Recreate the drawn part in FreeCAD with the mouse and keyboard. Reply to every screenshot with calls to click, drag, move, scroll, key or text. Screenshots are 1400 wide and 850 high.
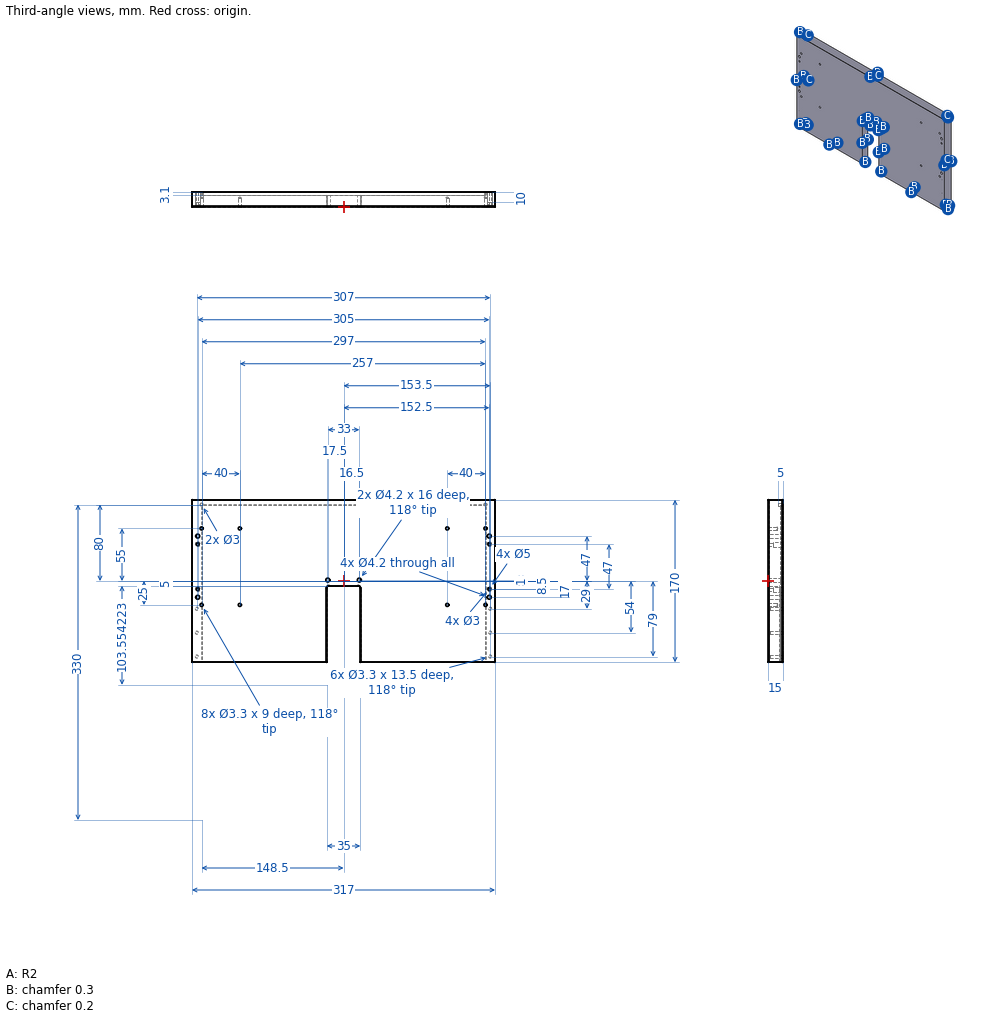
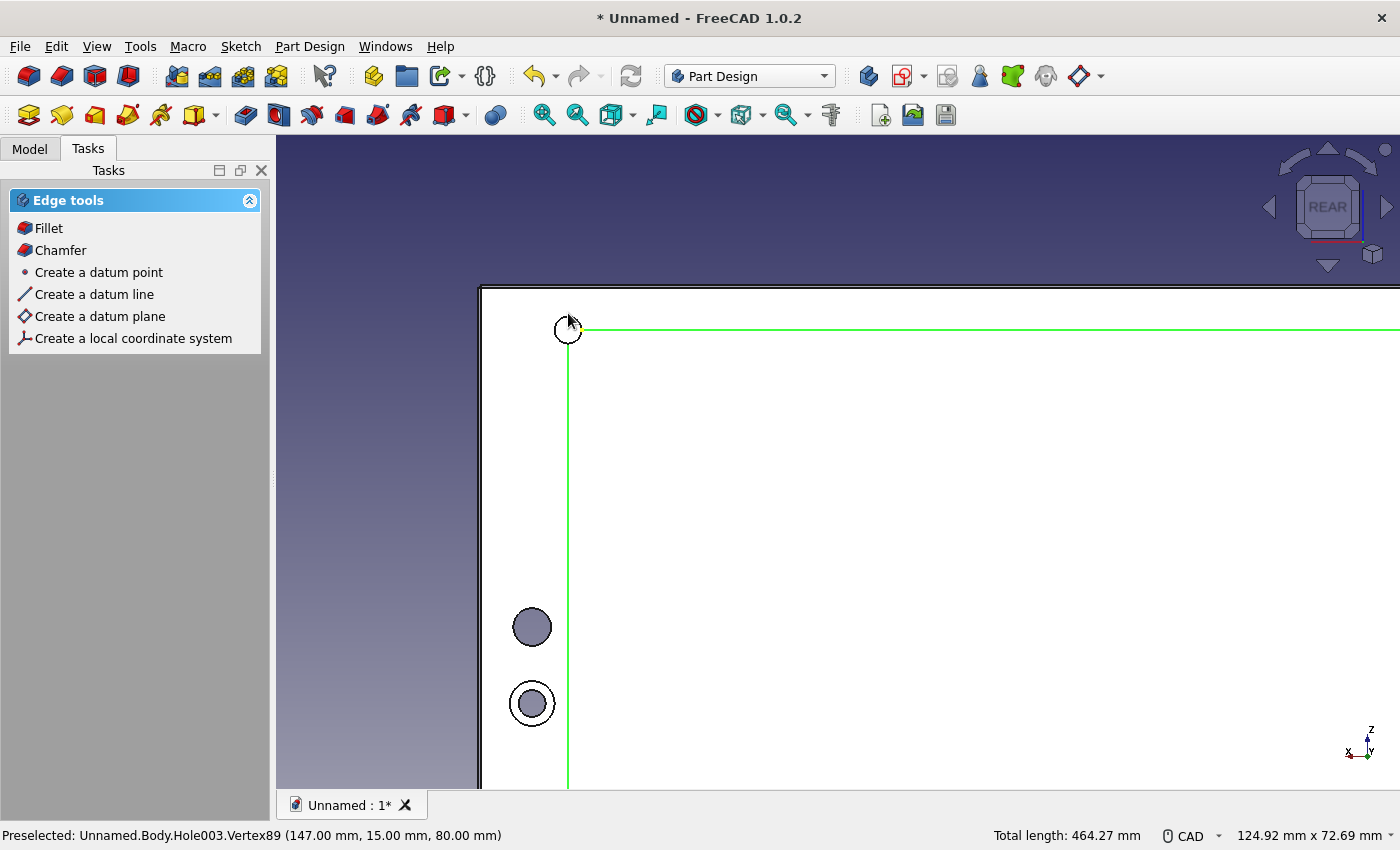
click(568, 316, ctrl)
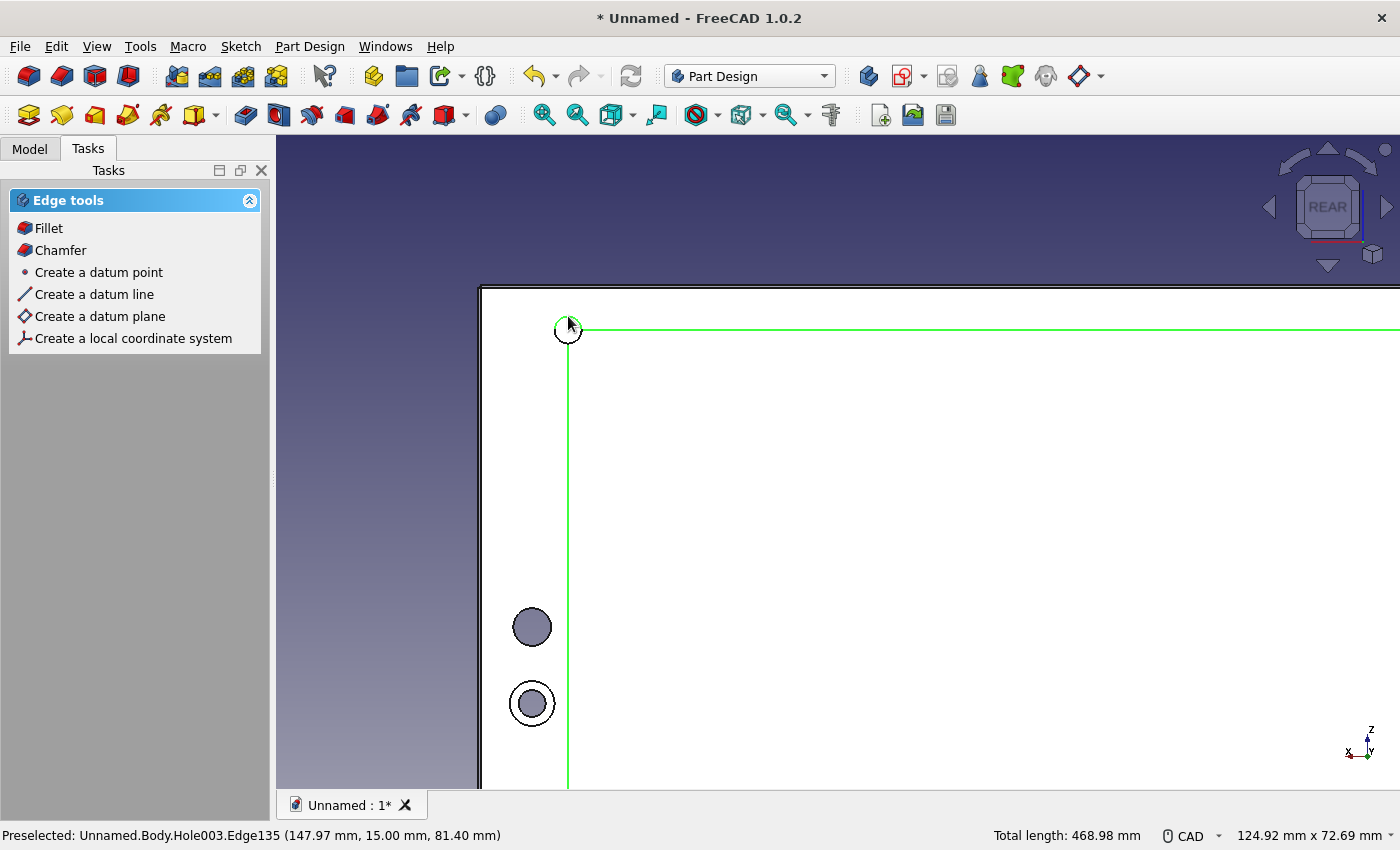
key(v)
key(f)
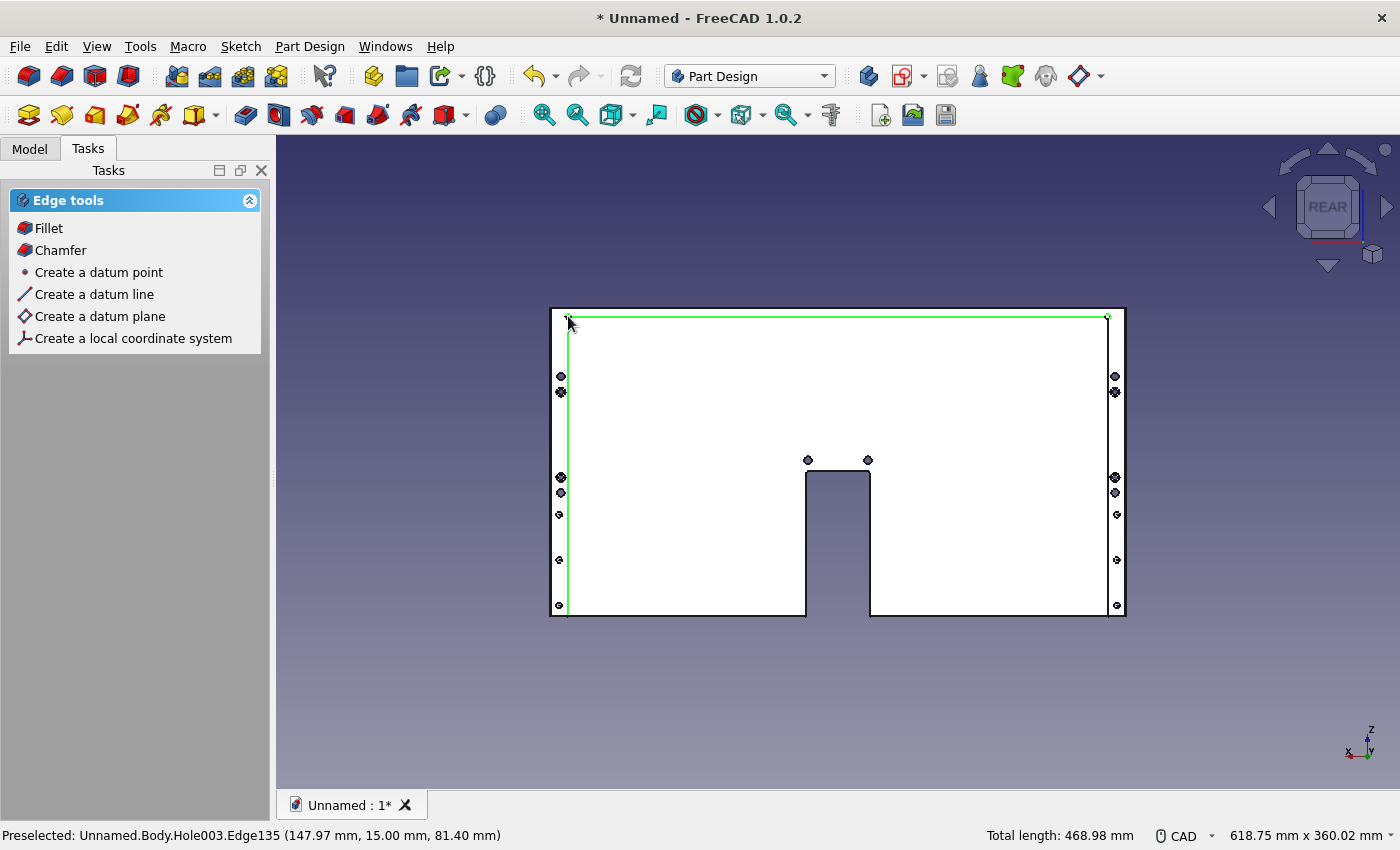
key(0)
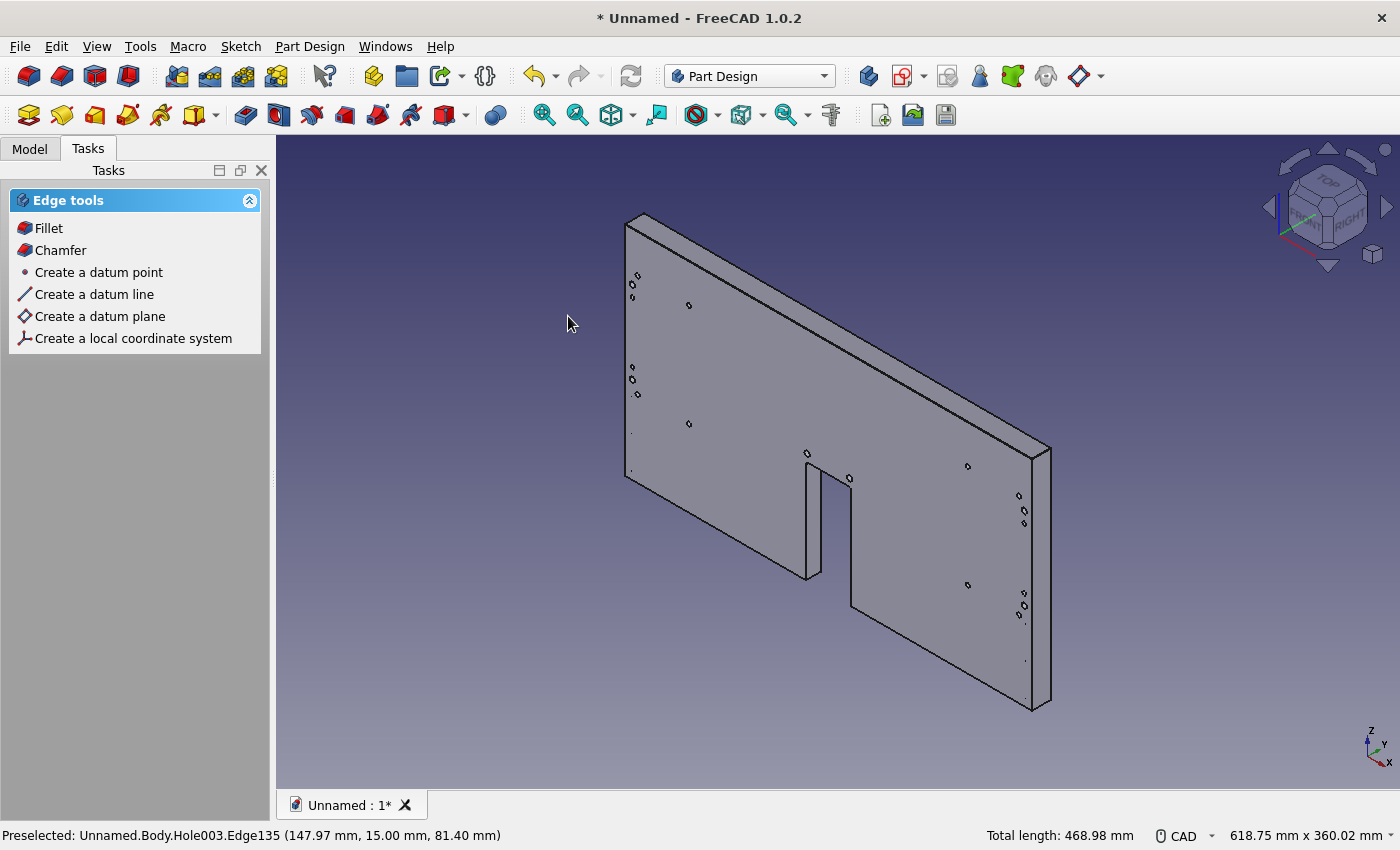
key(2)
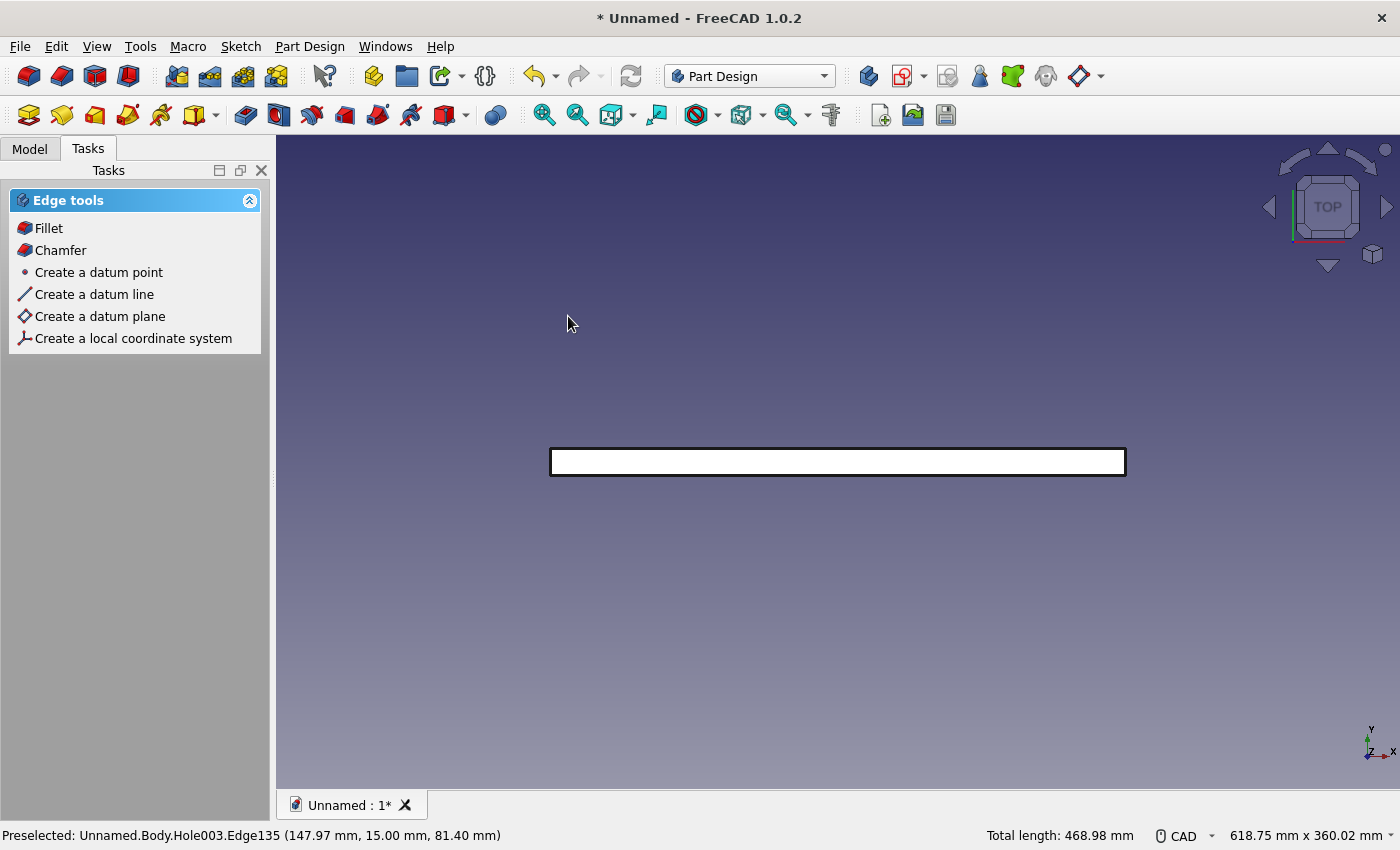
key(1)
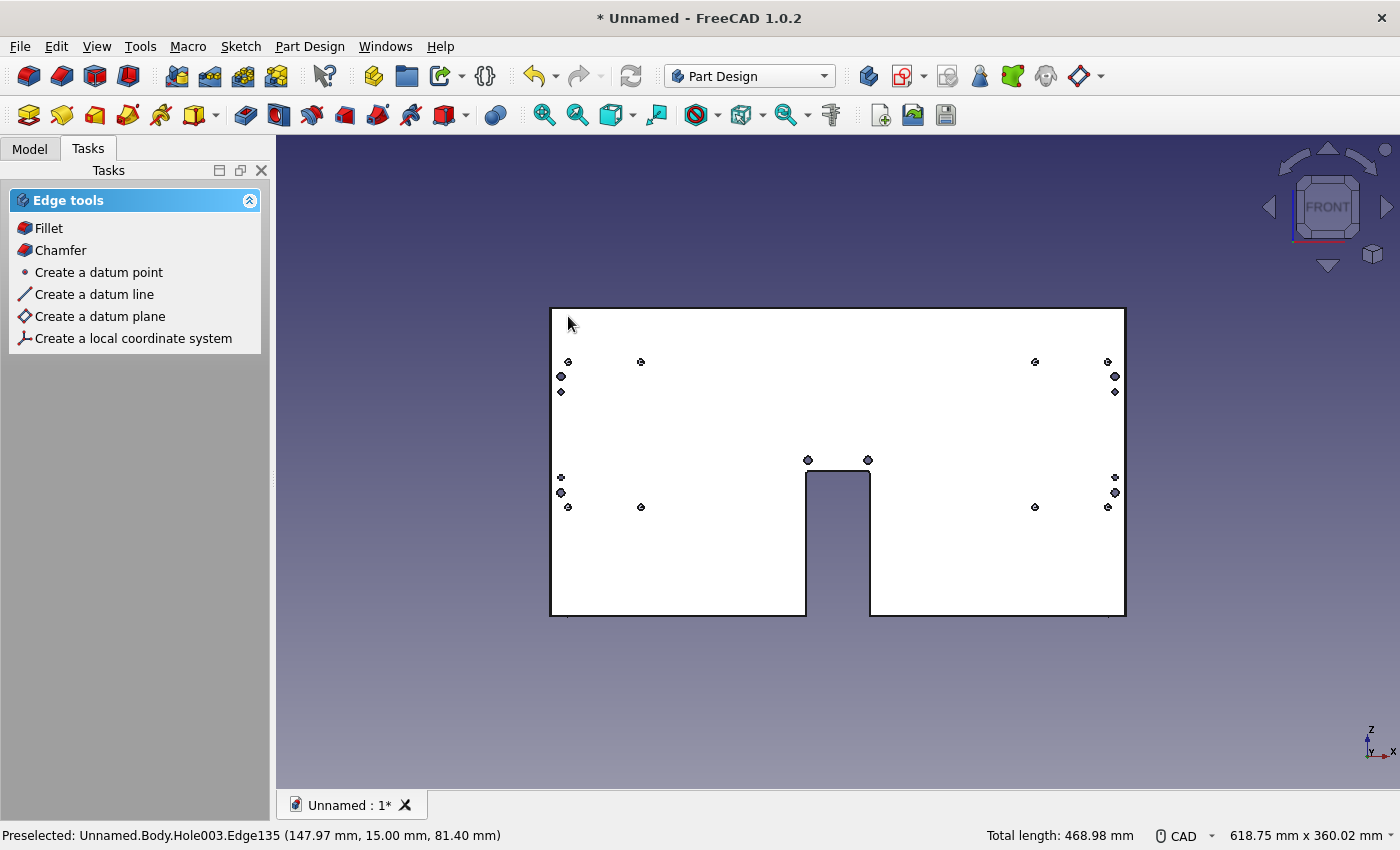
key(3)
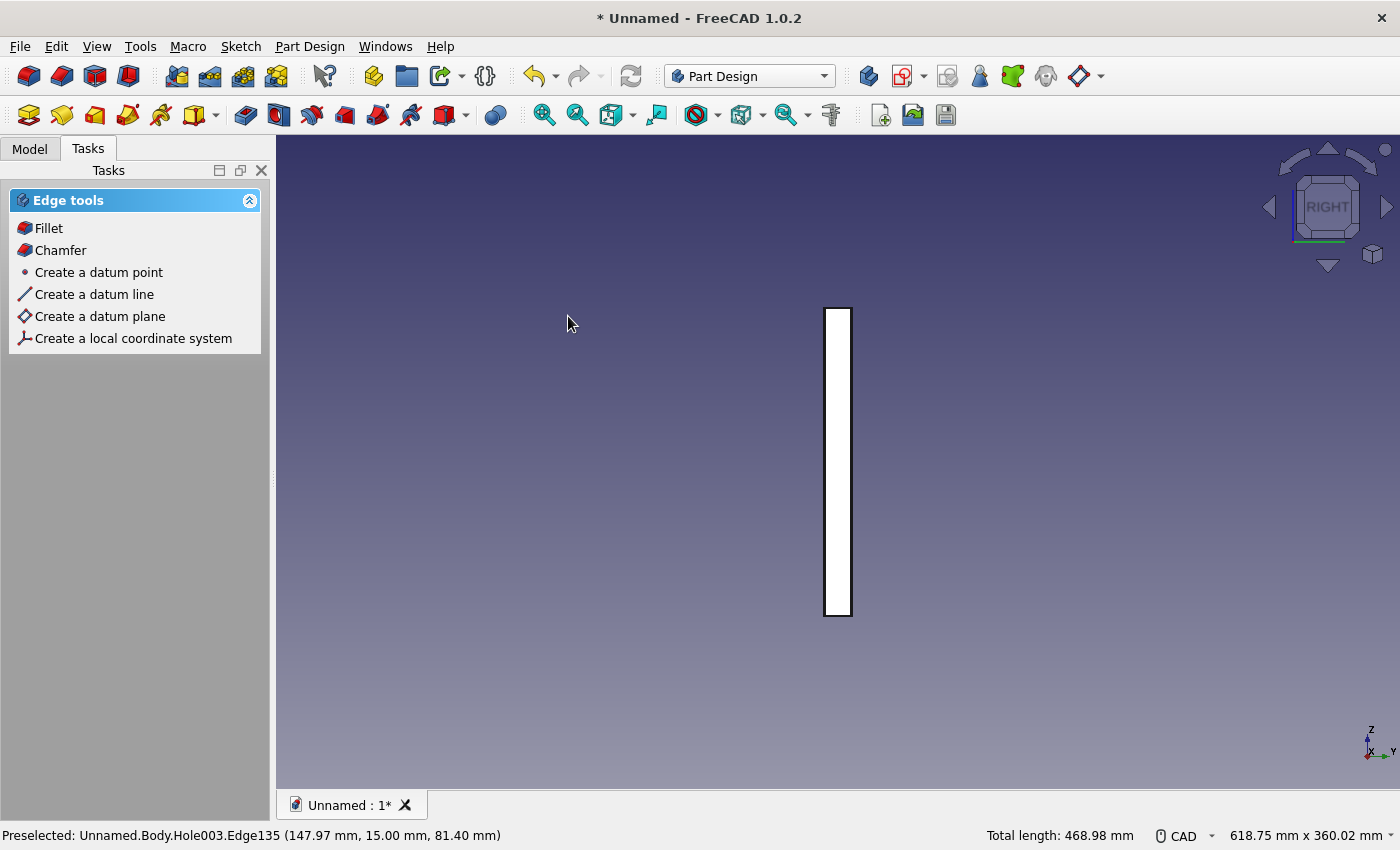
key(5)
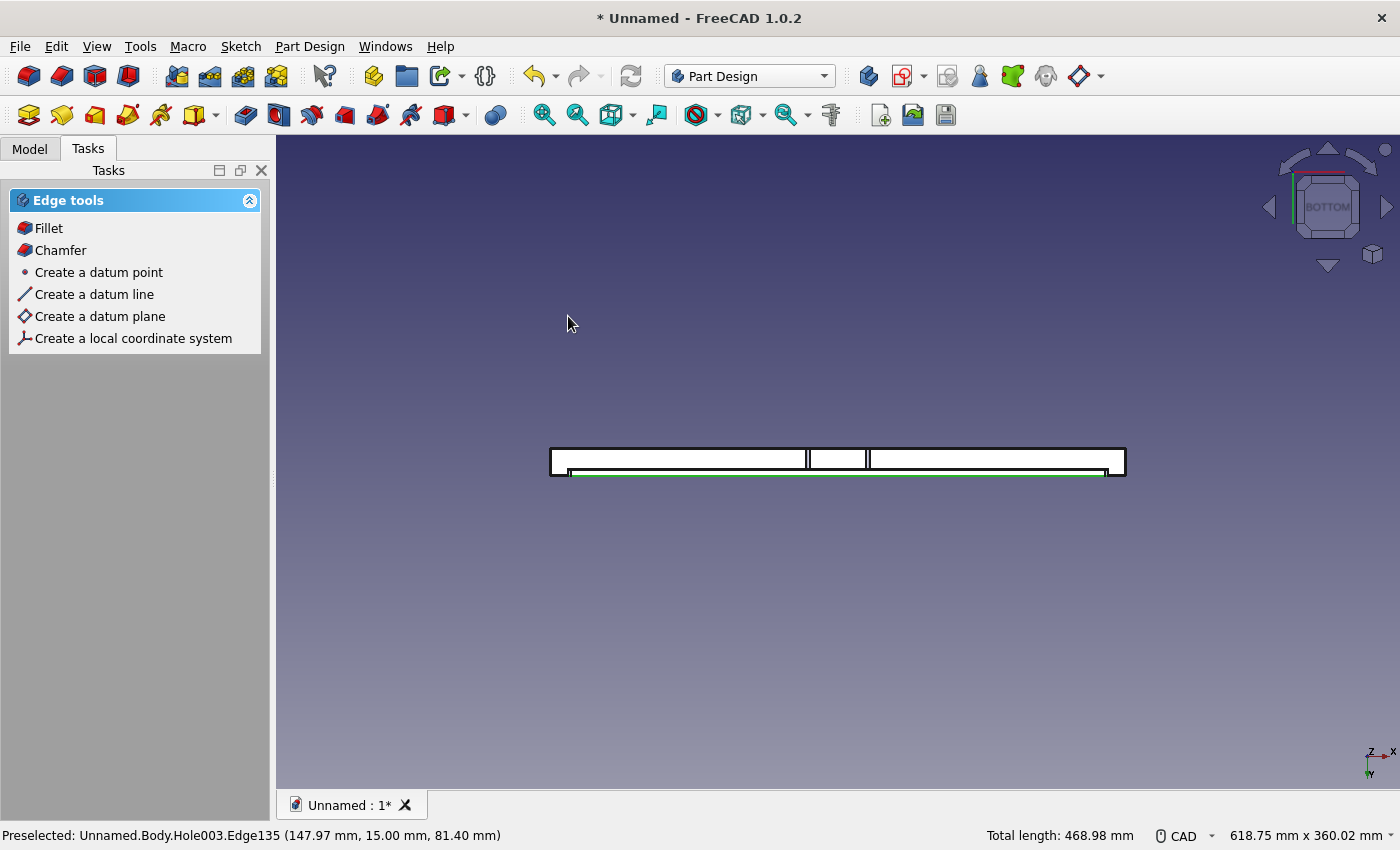
key(4)